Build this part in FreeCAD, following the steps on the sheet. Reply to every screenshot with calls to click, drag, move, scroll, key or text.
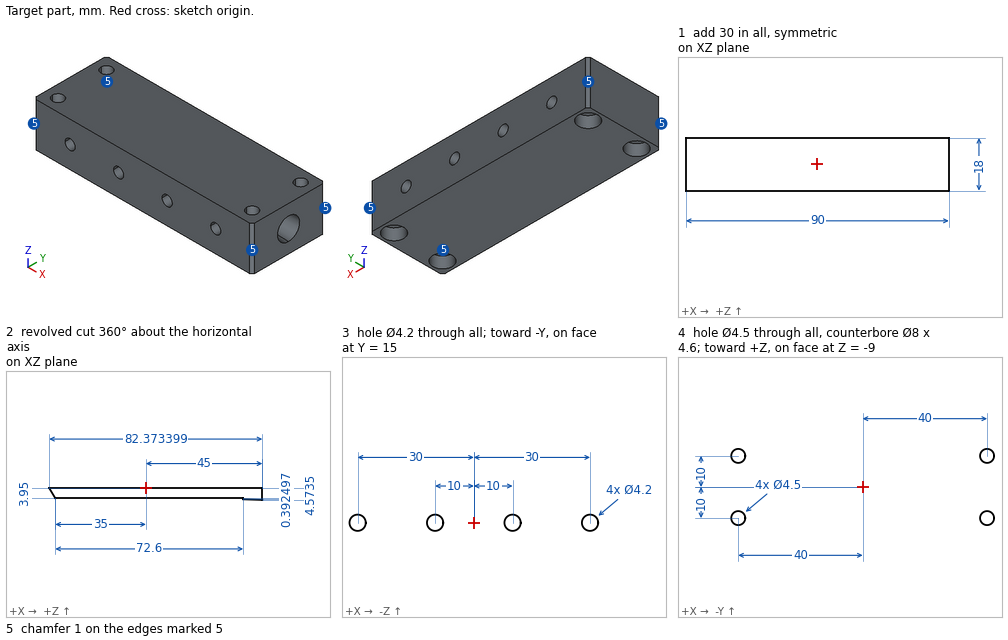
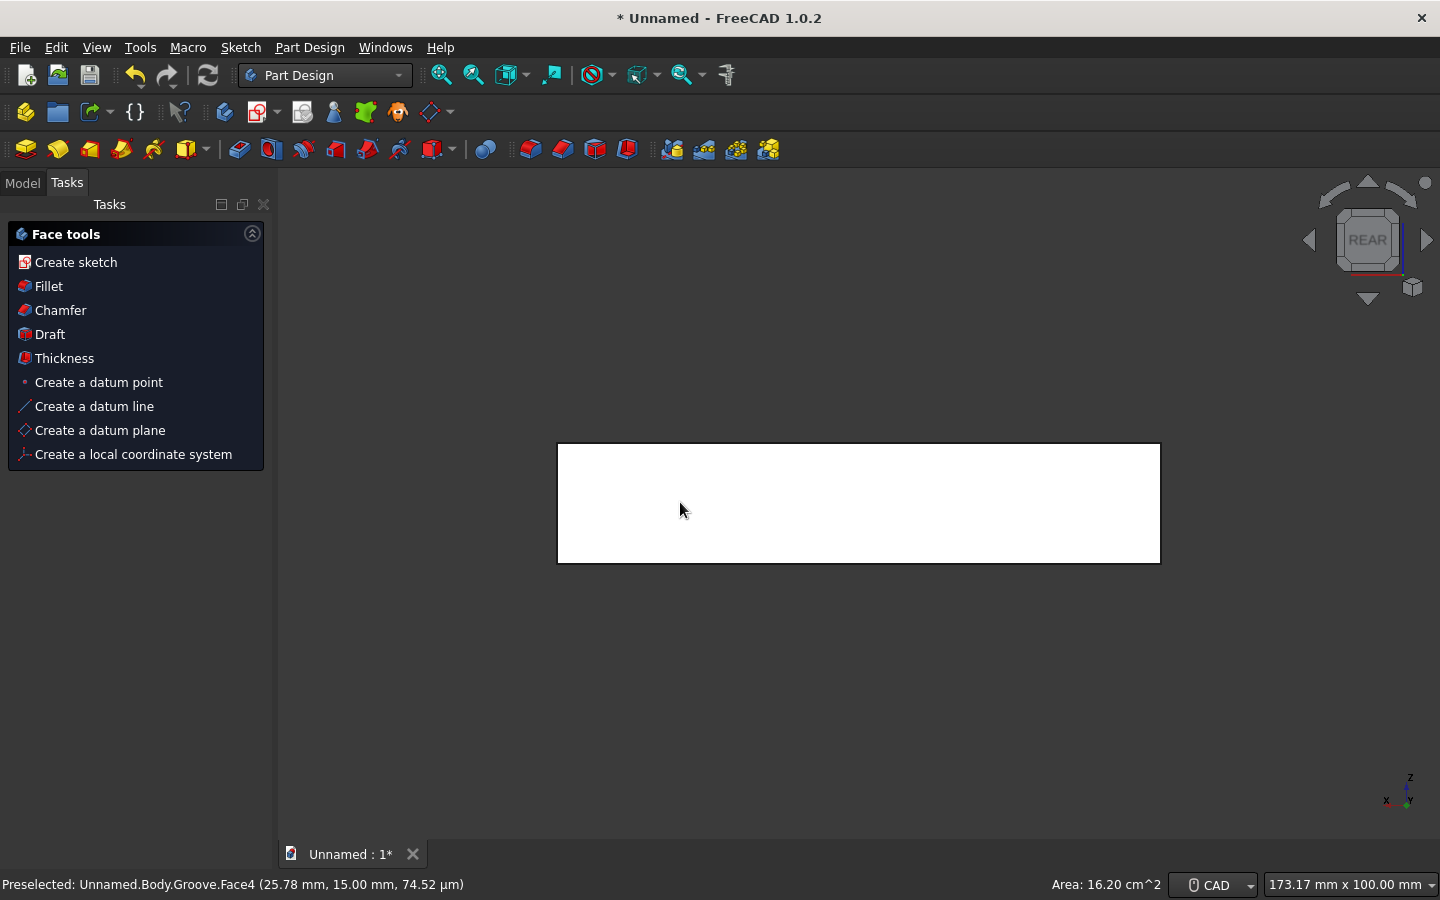
click(258, 112)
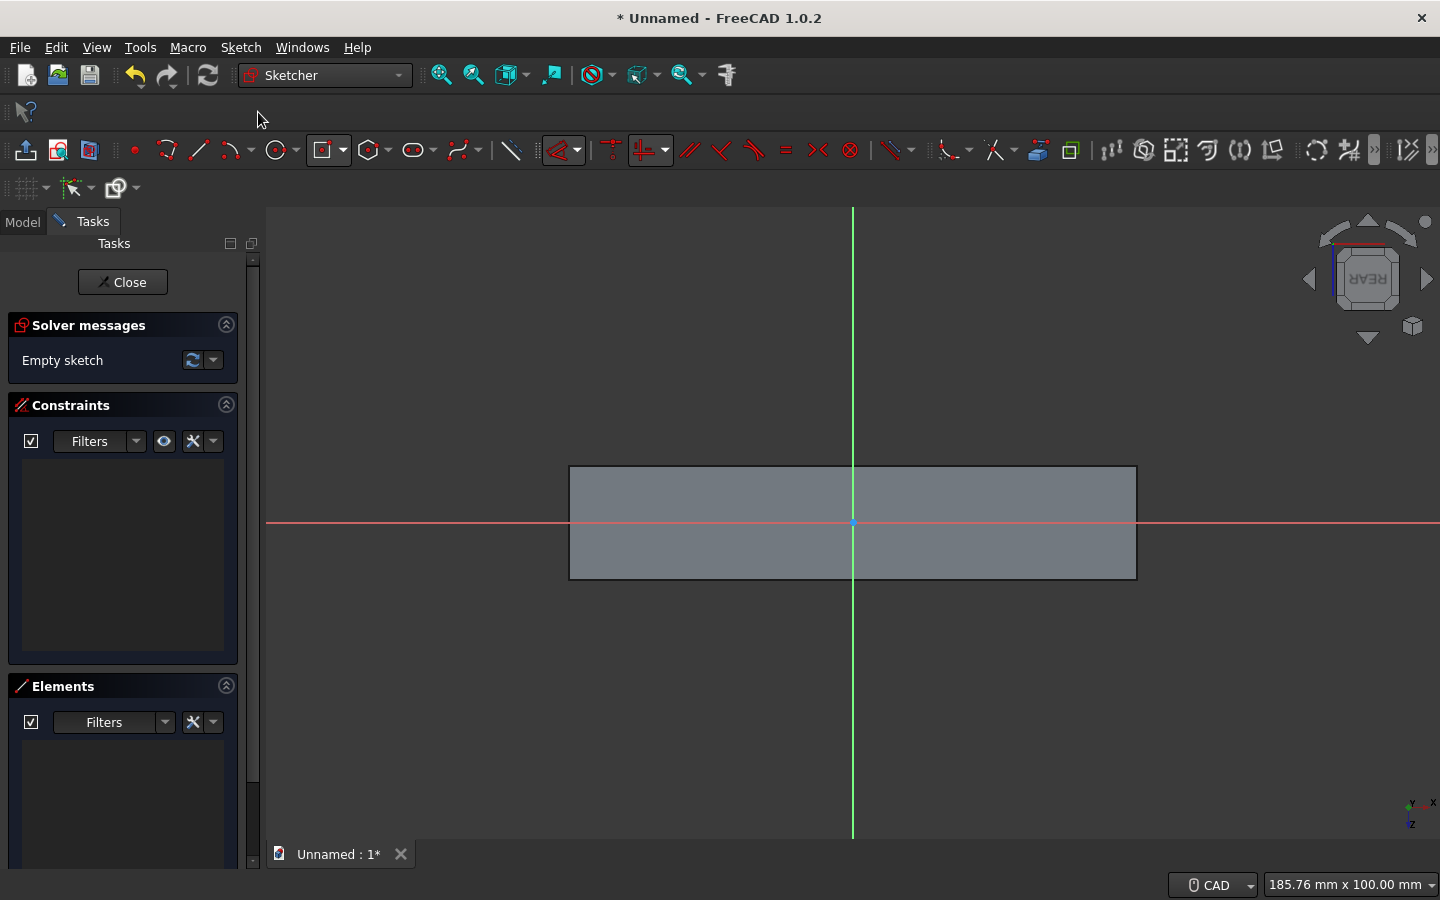
scroll(936, 523, up, 3)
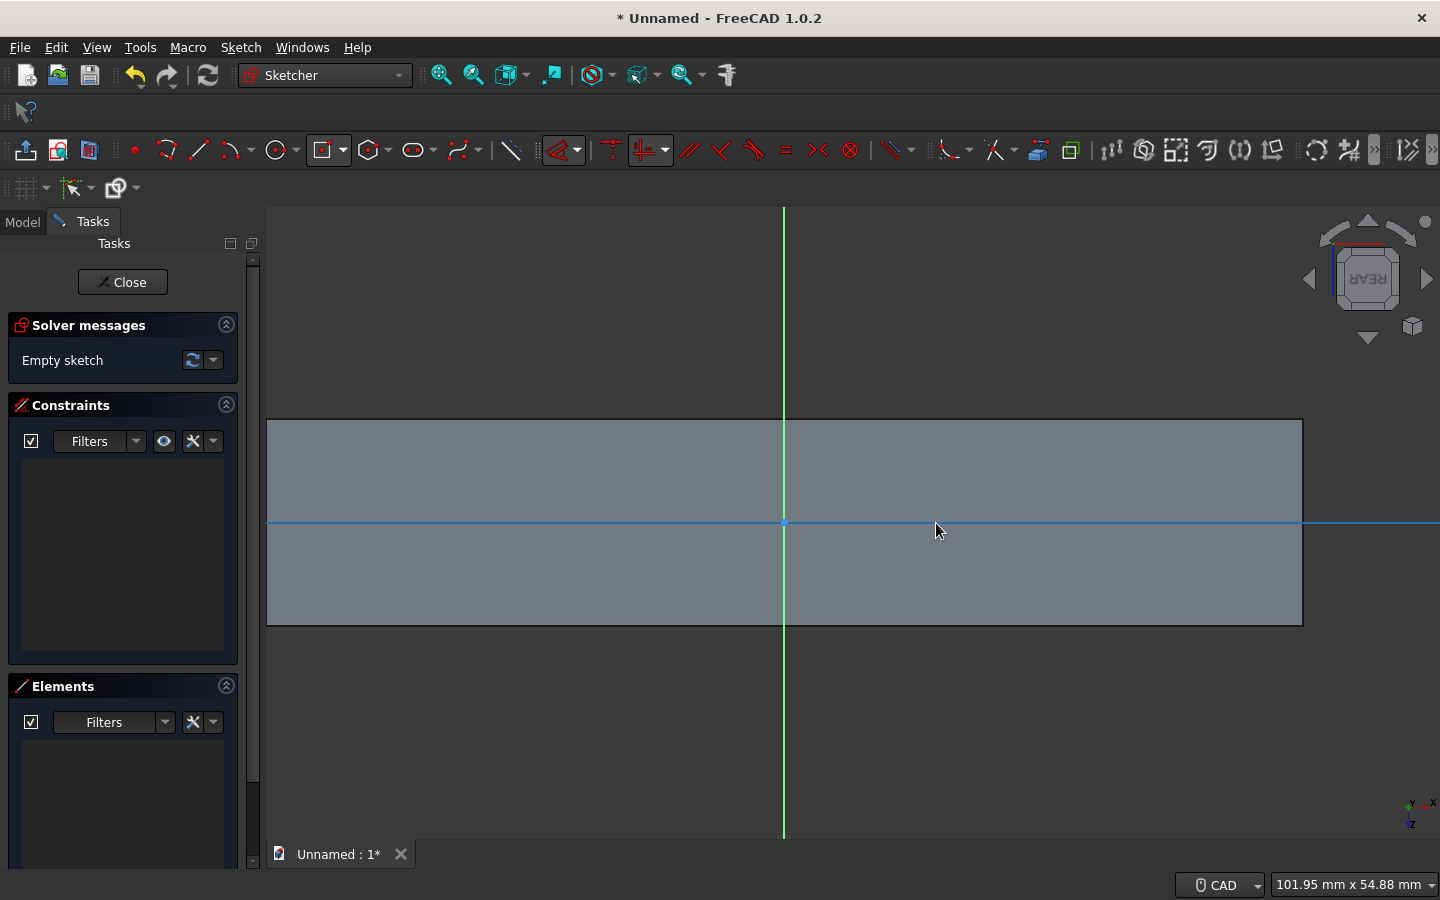
click(276, 150)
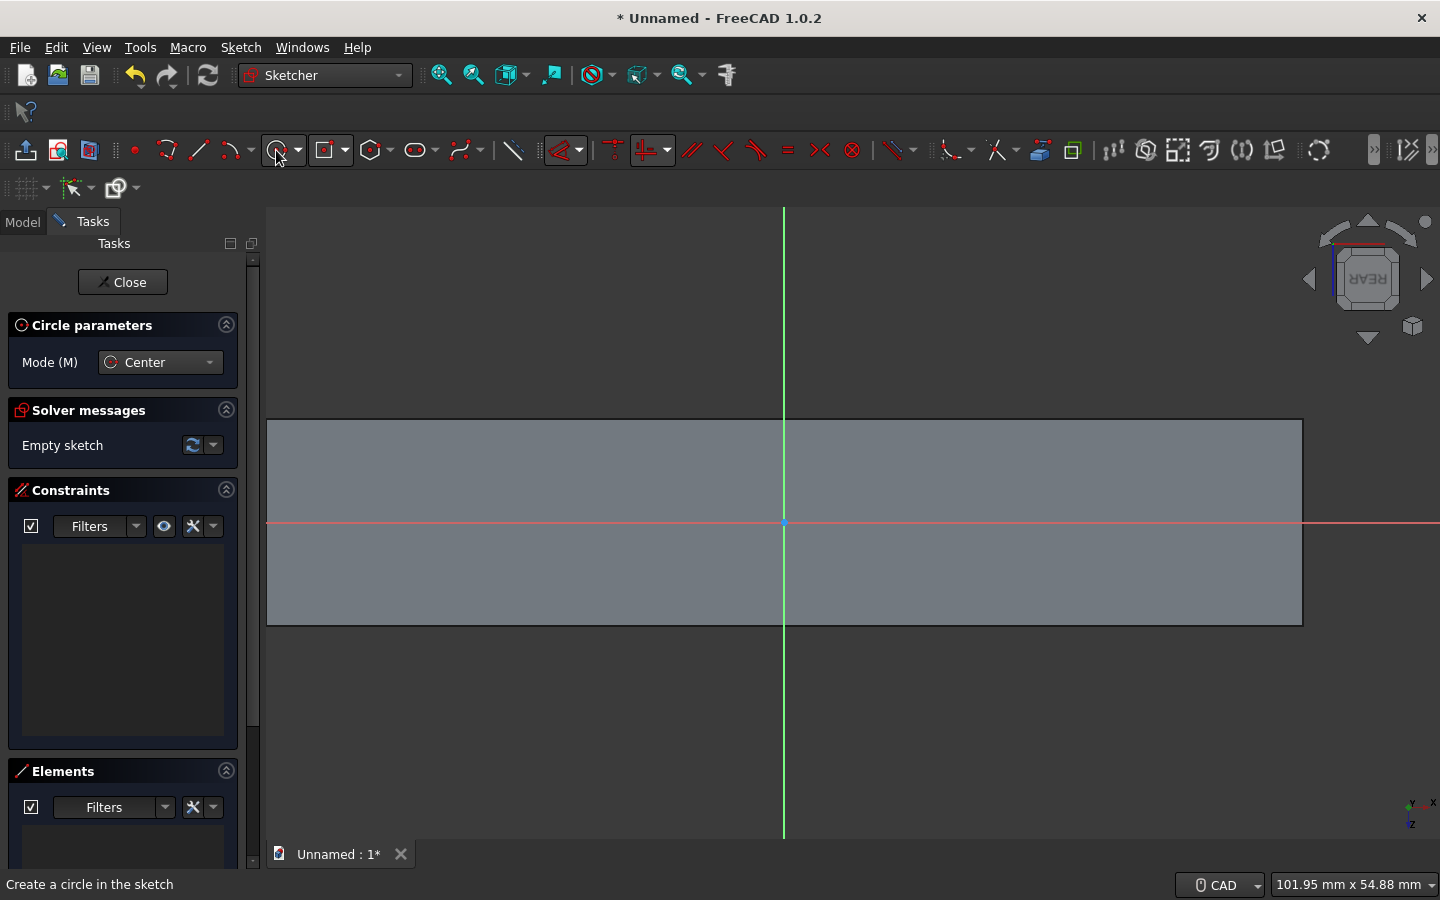
click(1130, 523)
click(1147, 505)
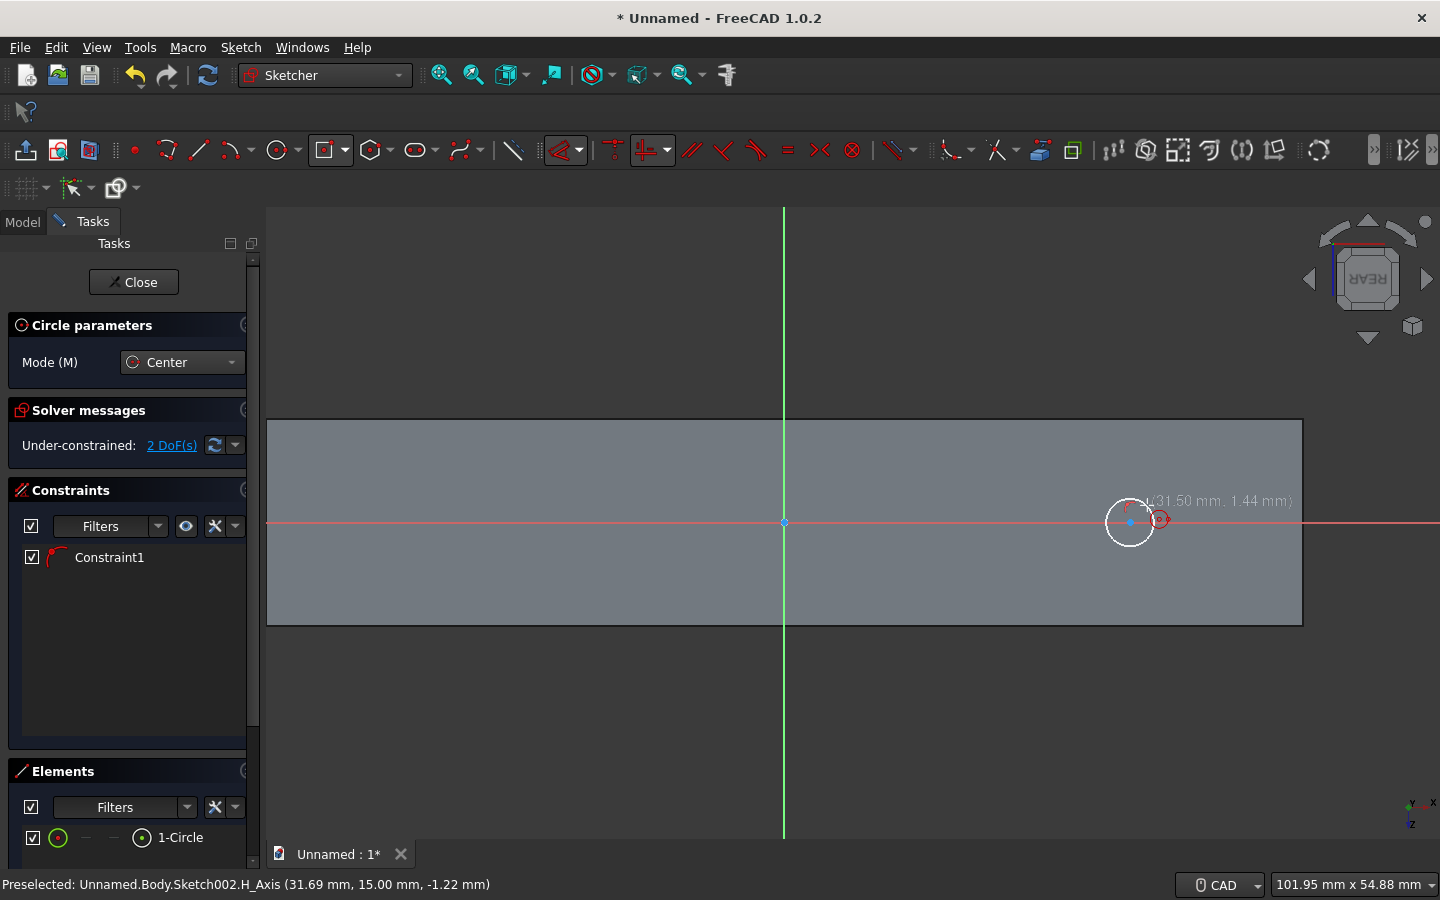
click(899, 523)
click(917, 505)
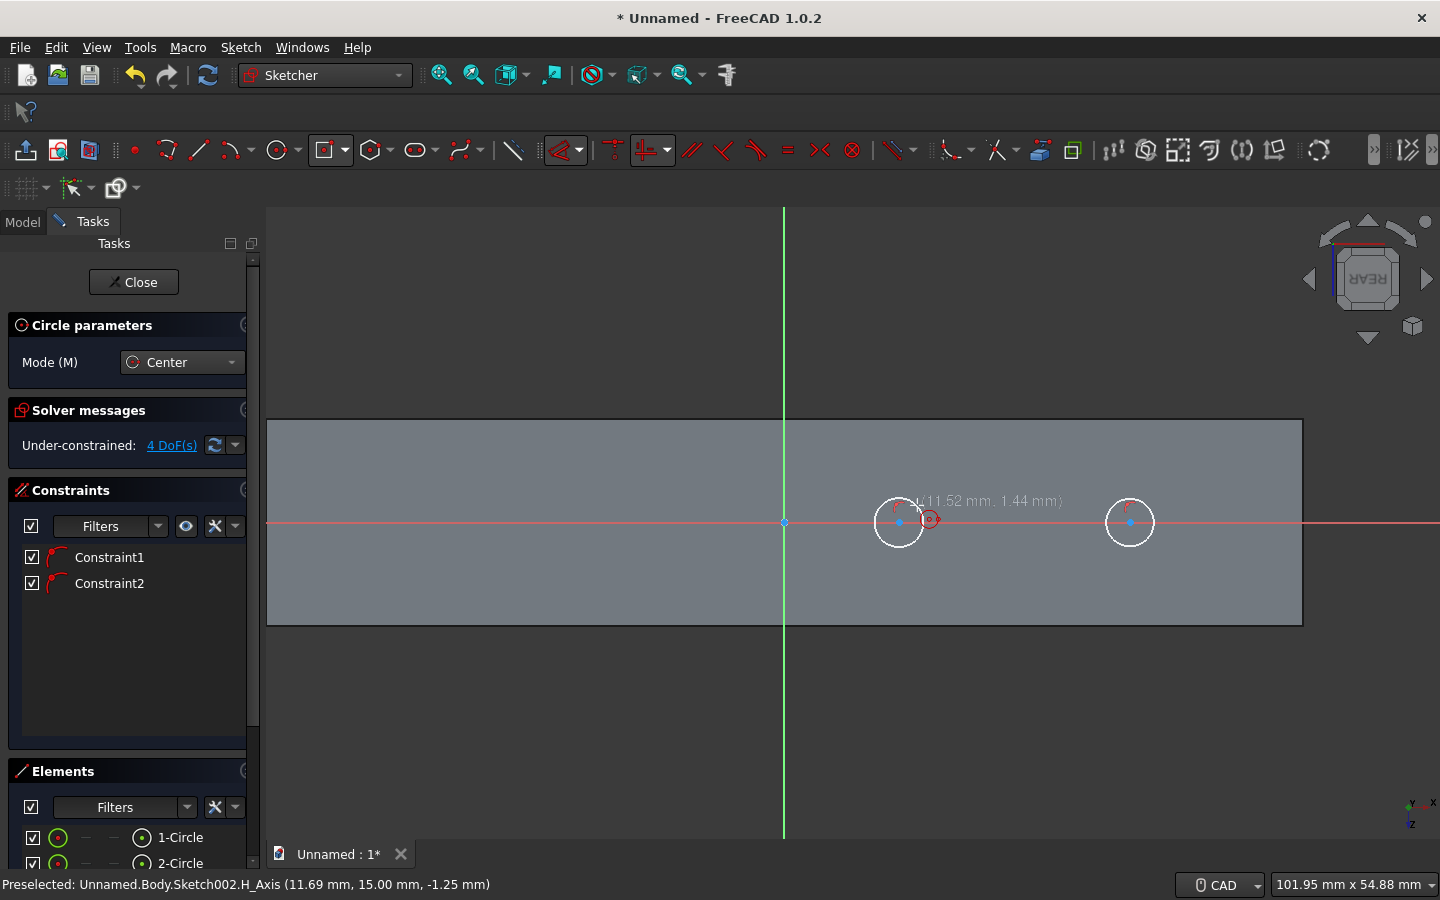
click(669, 523)
click(686, 505)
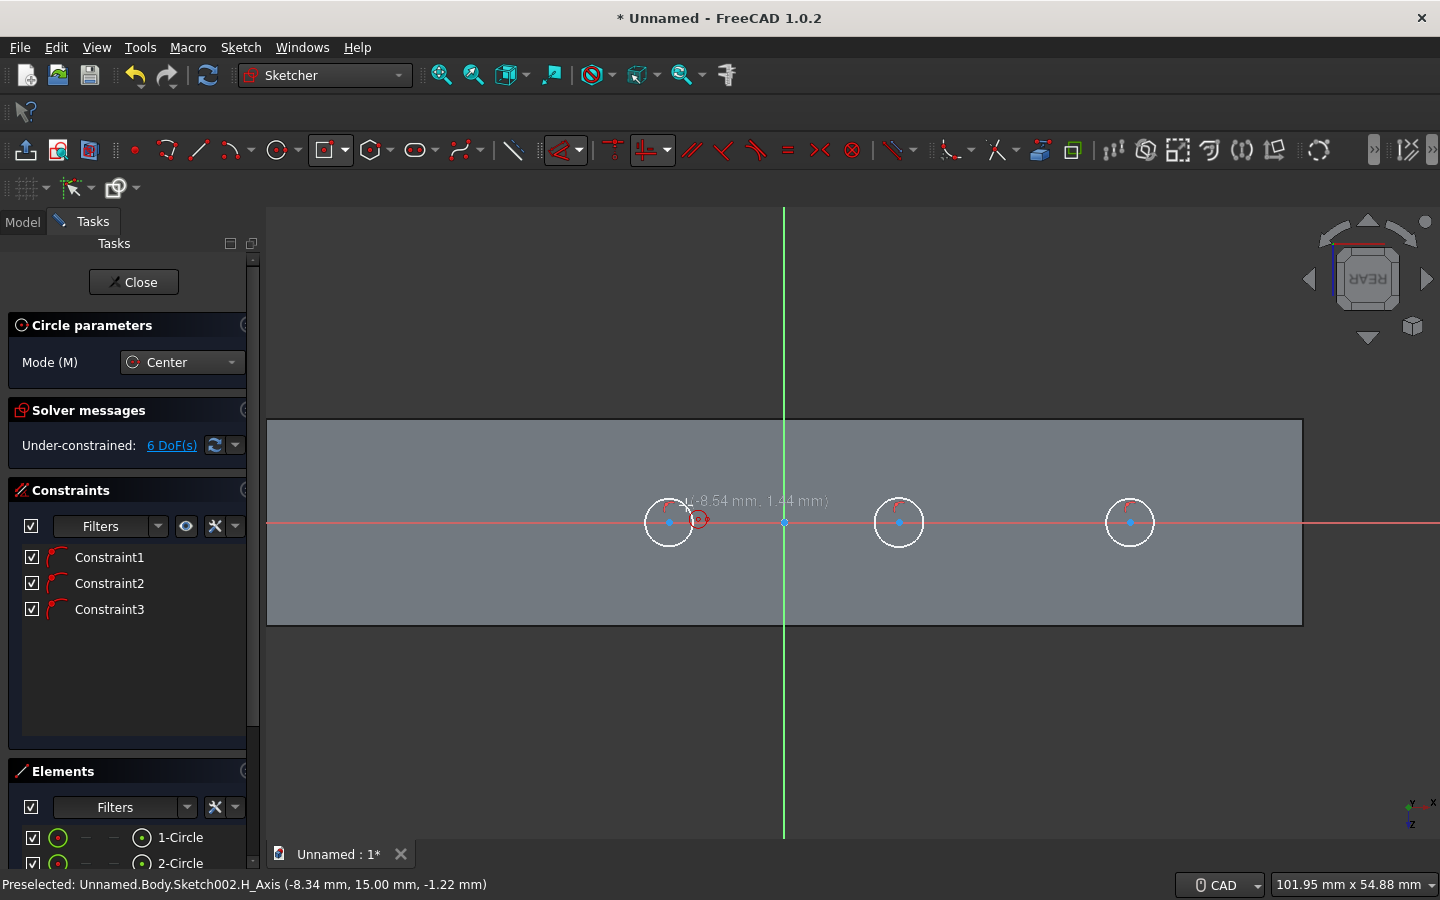
click(439, 523)
click(456, 505)
key(Escape)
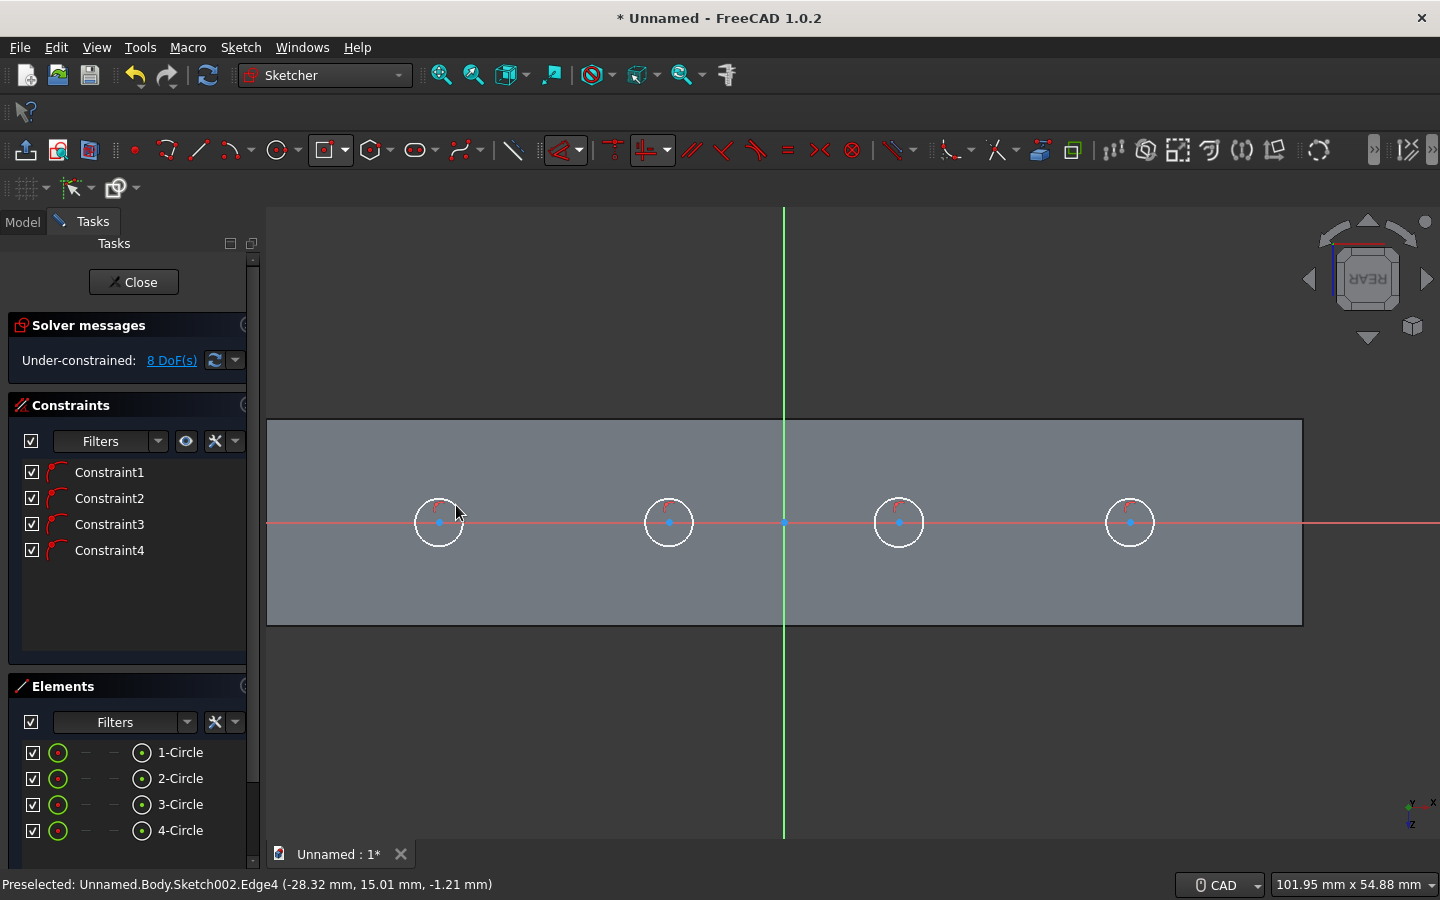
click(1147, 506)